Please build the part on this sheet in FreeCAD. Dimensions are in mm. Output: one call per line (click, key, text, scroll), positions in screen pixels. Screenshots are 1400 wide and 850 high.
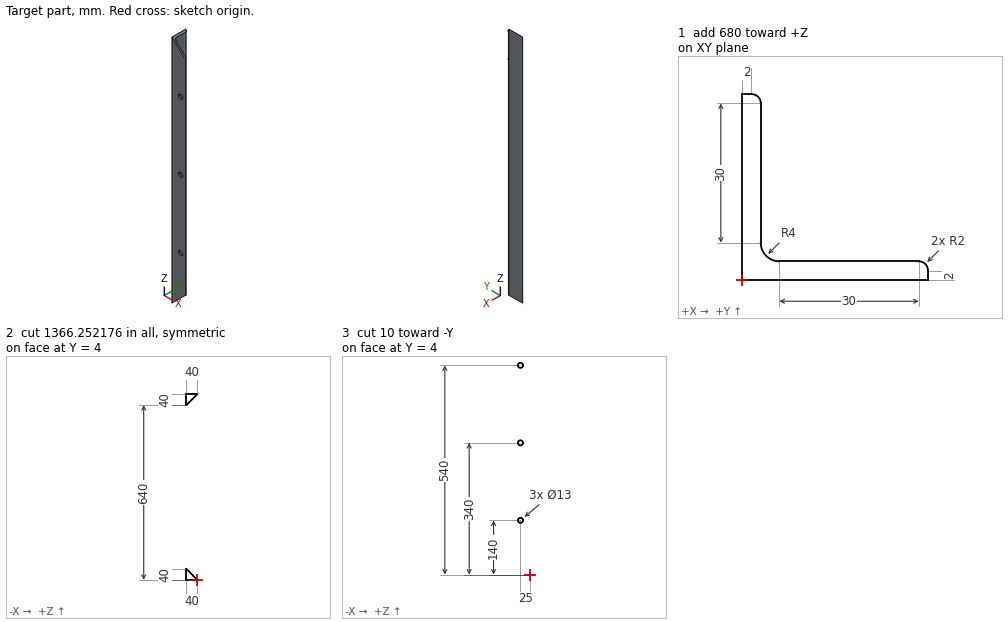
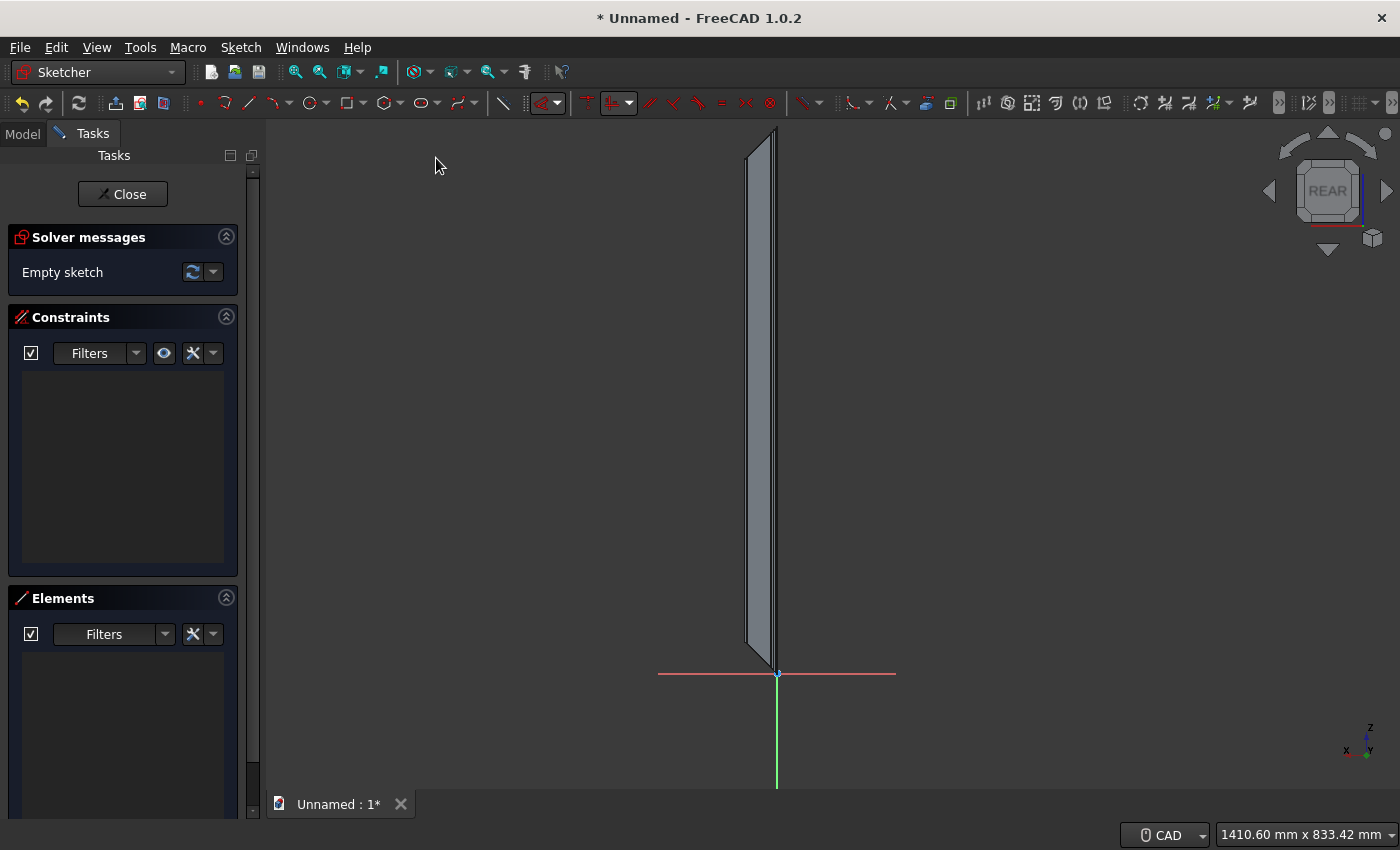
click(310, 104)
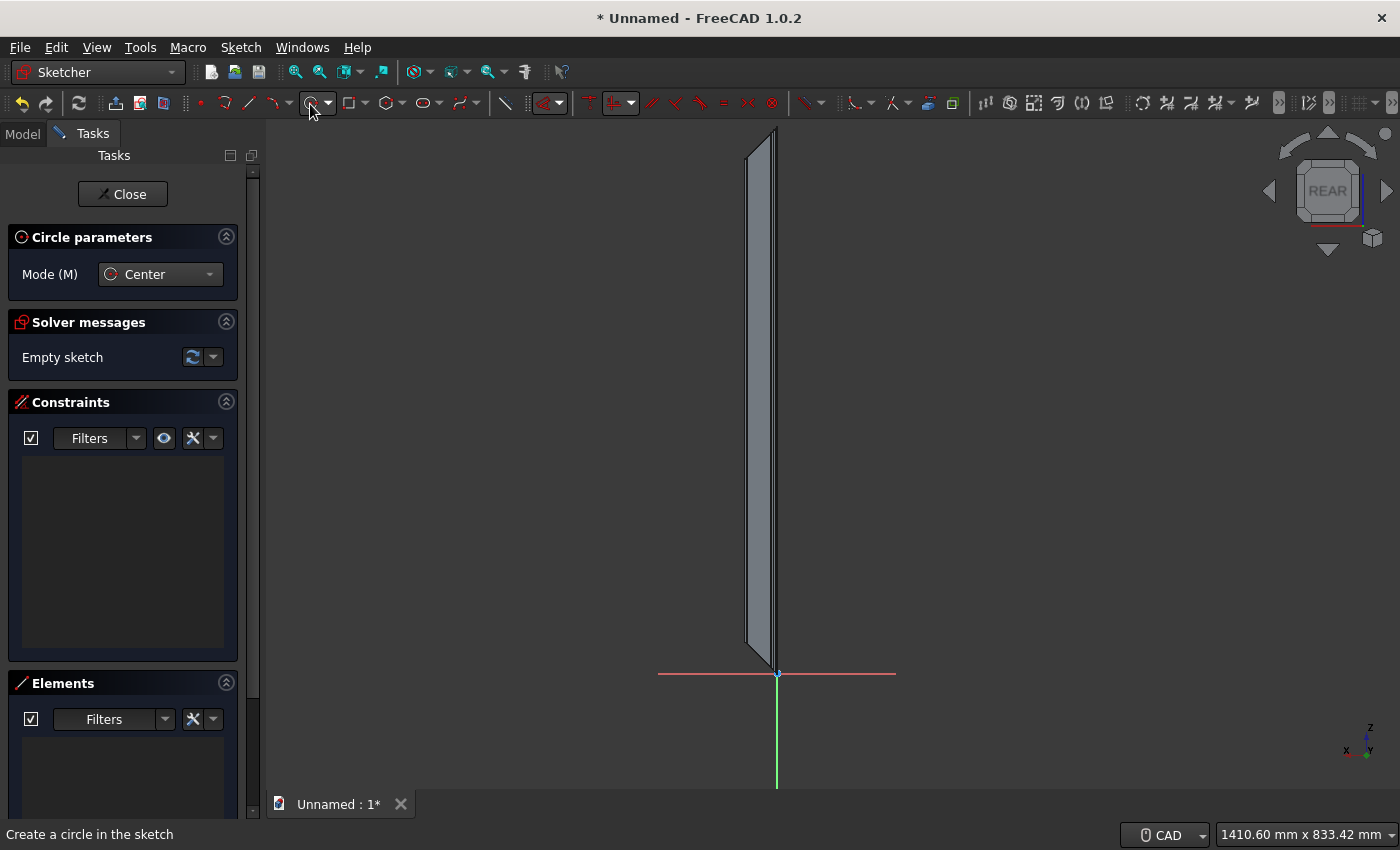
scroll(757, 561, up, 8)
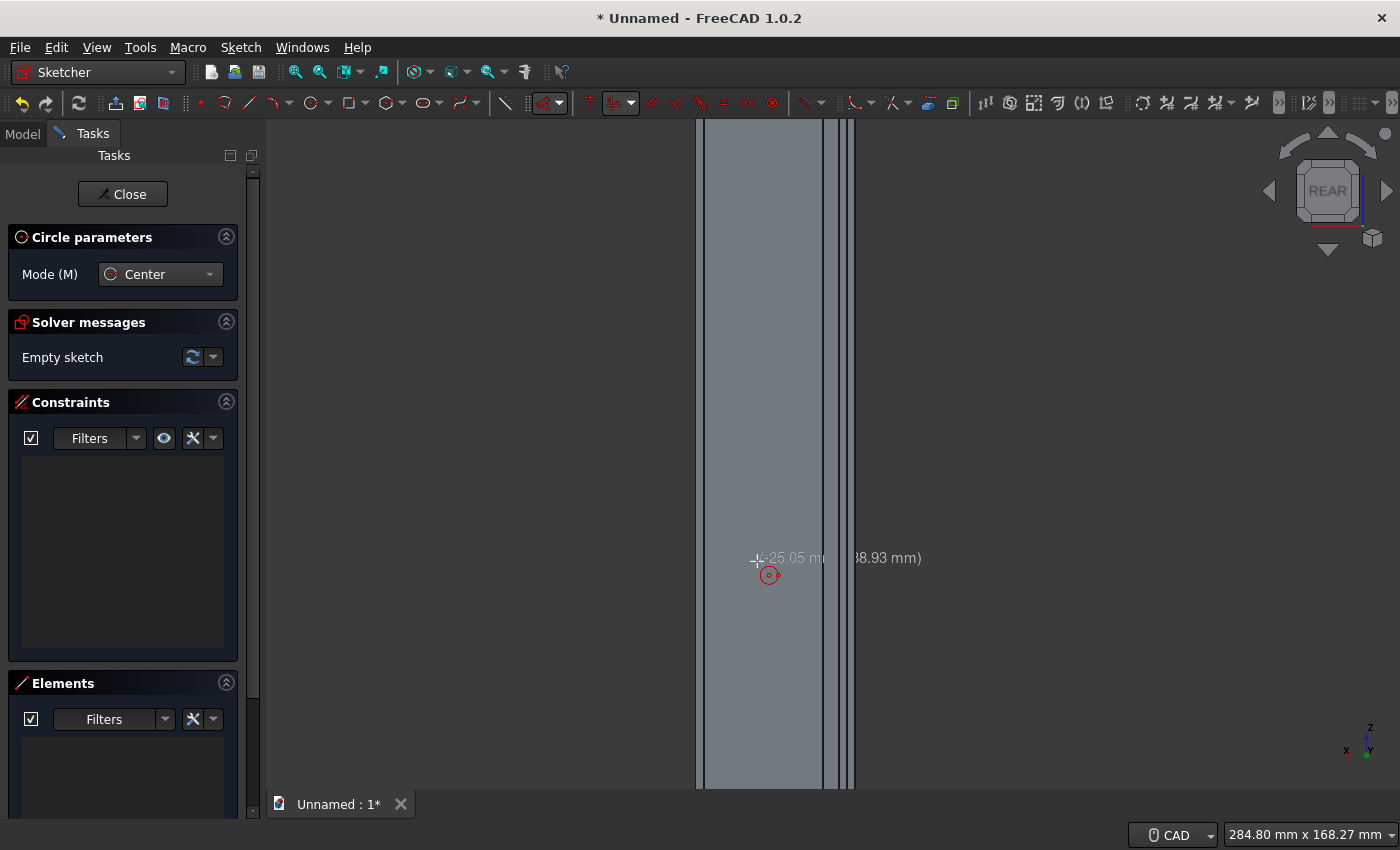
scroll(757, 562, down, 8)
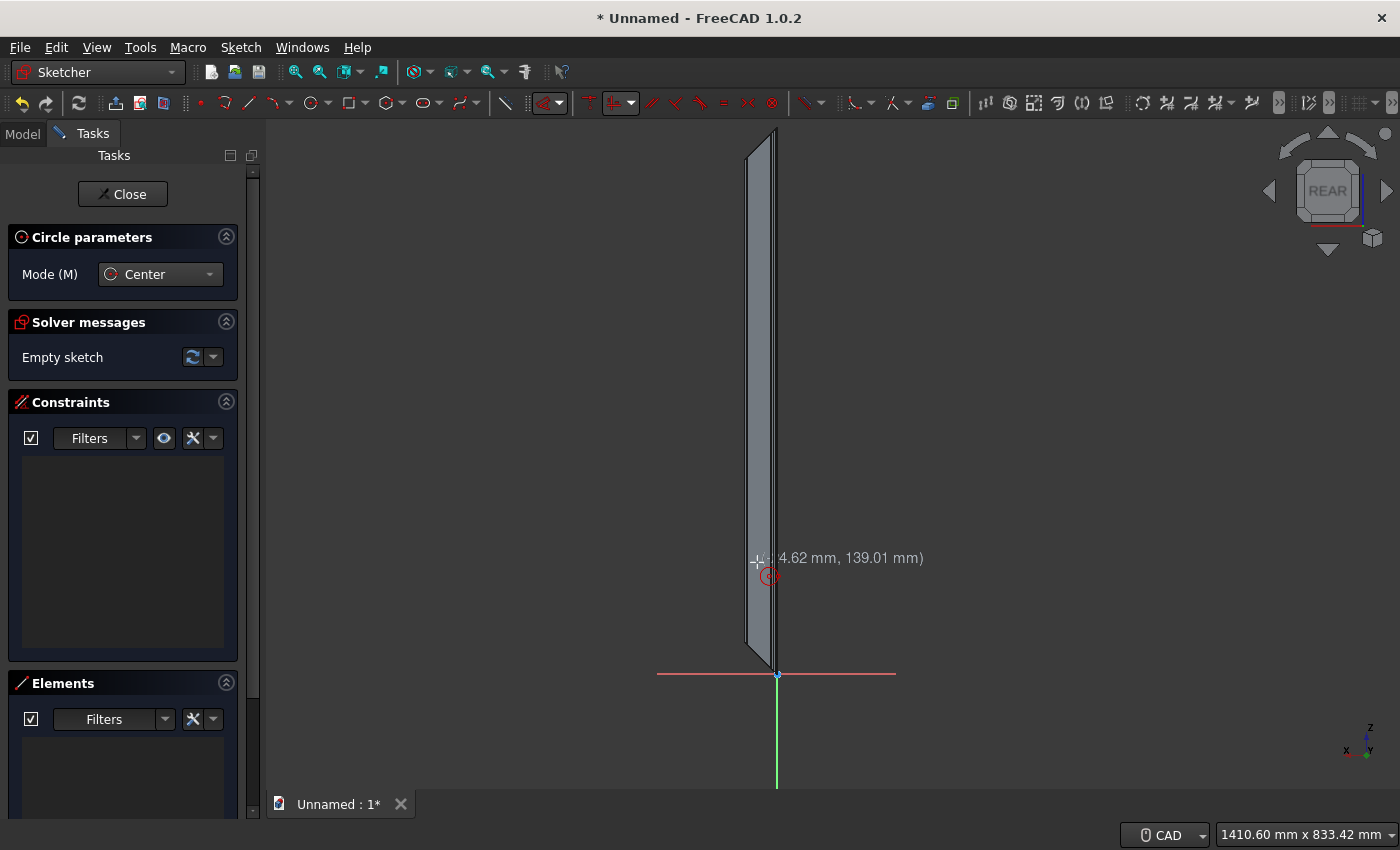
click(757, 562)
move(761, 558)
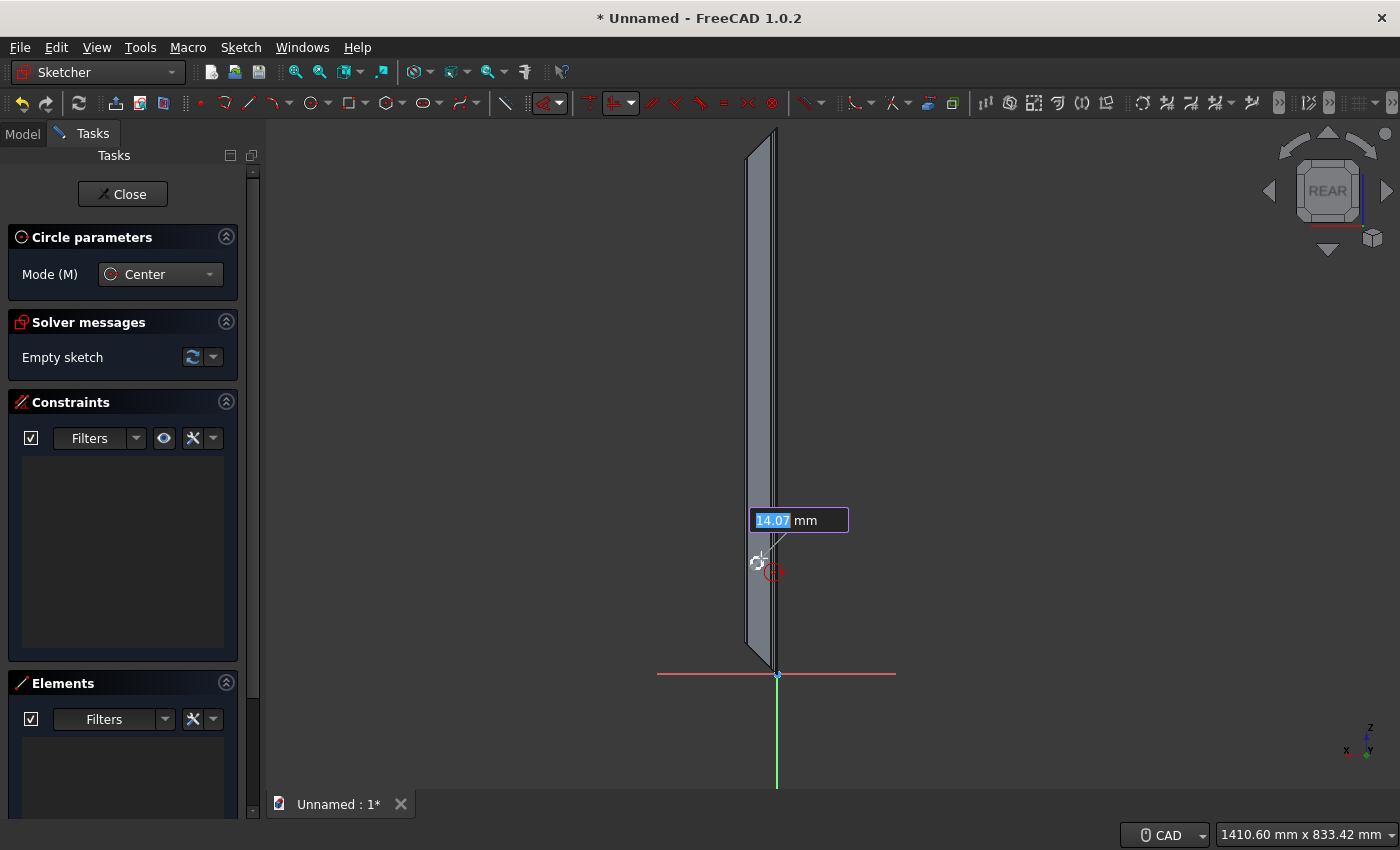
text(13)
key(Return)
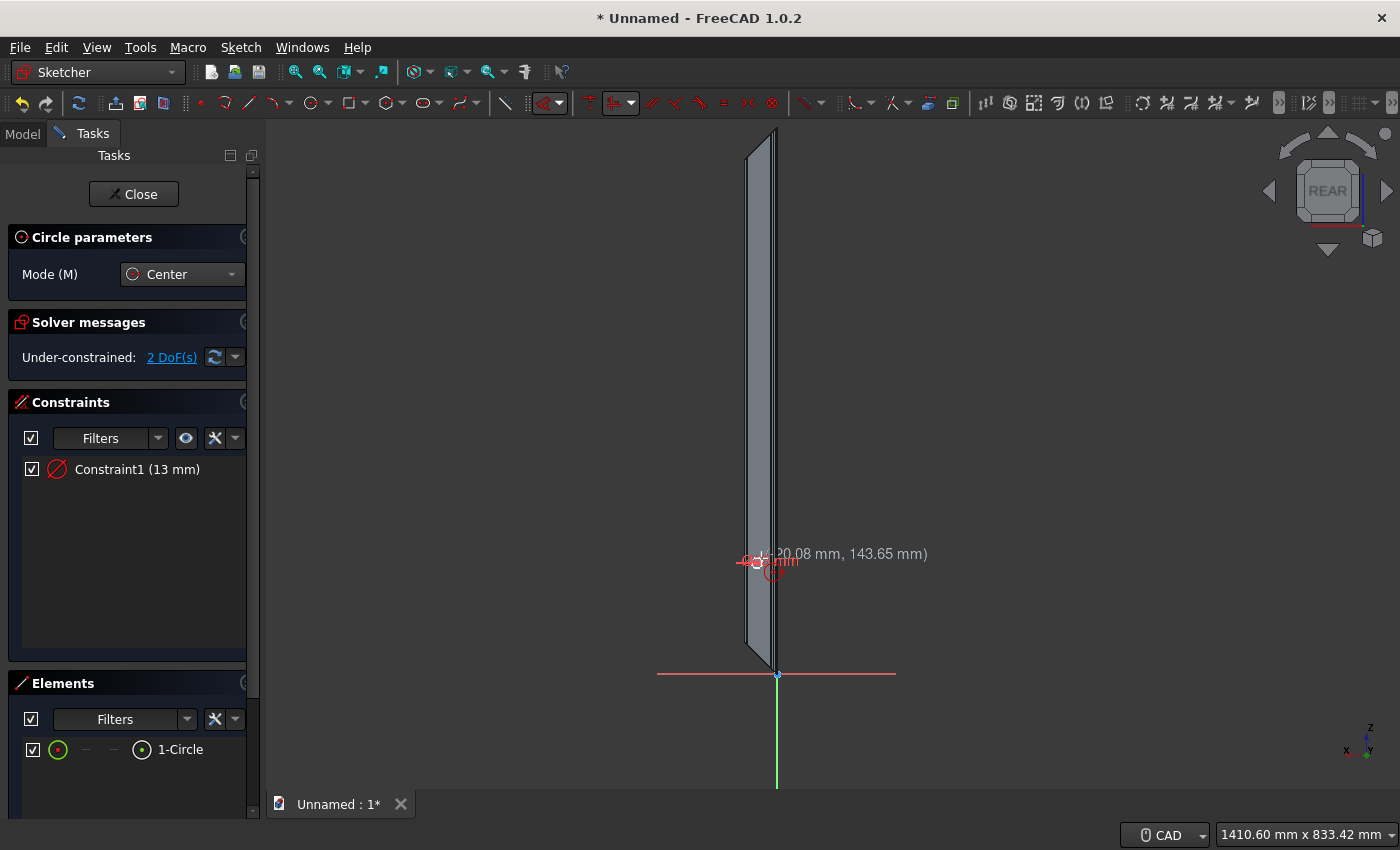
scroll(757, 401, up, 8)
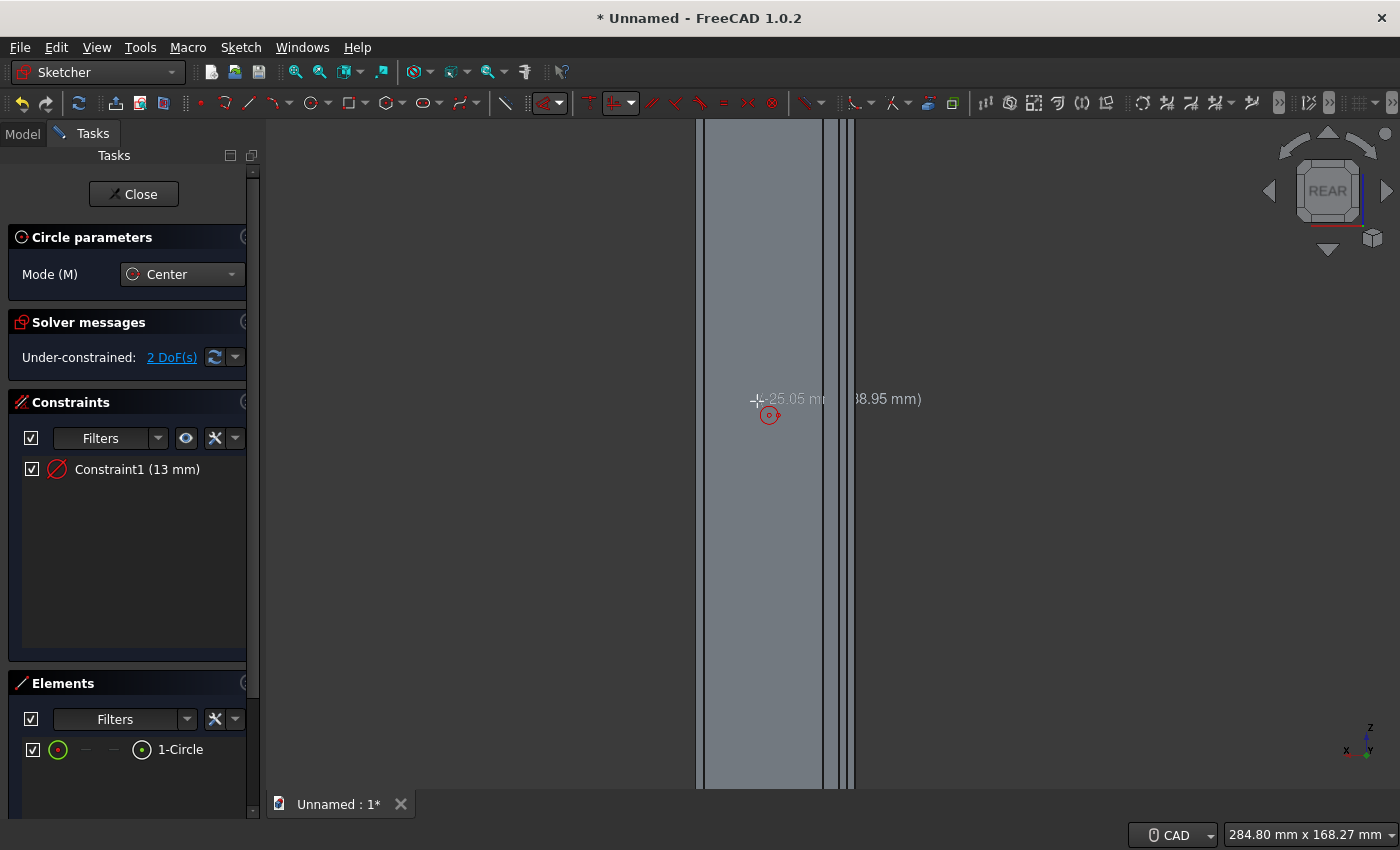
scroll(757, 400, down, 8)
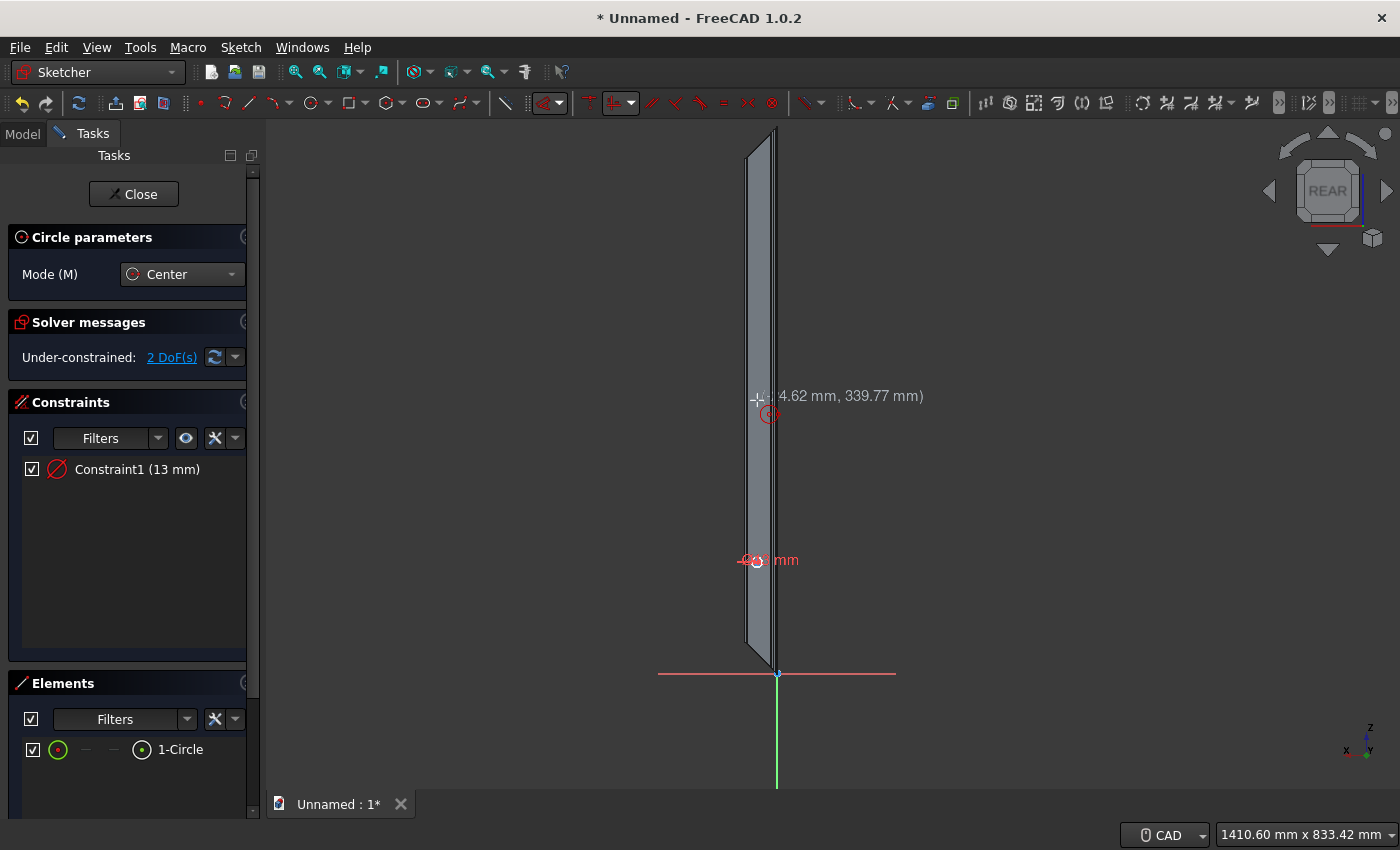
click(757, 400)
move(761, 397)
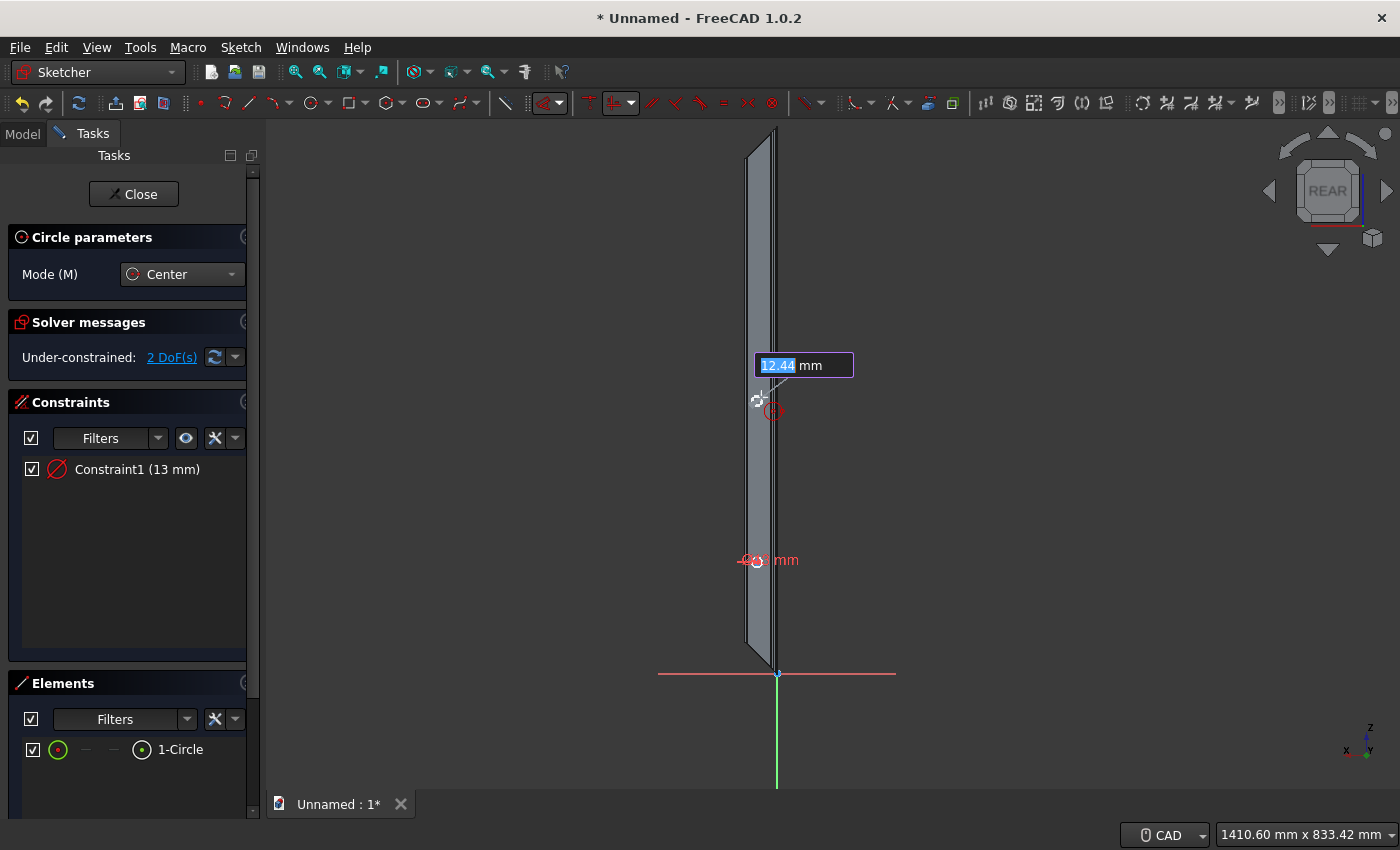
text(13)
key(Return)